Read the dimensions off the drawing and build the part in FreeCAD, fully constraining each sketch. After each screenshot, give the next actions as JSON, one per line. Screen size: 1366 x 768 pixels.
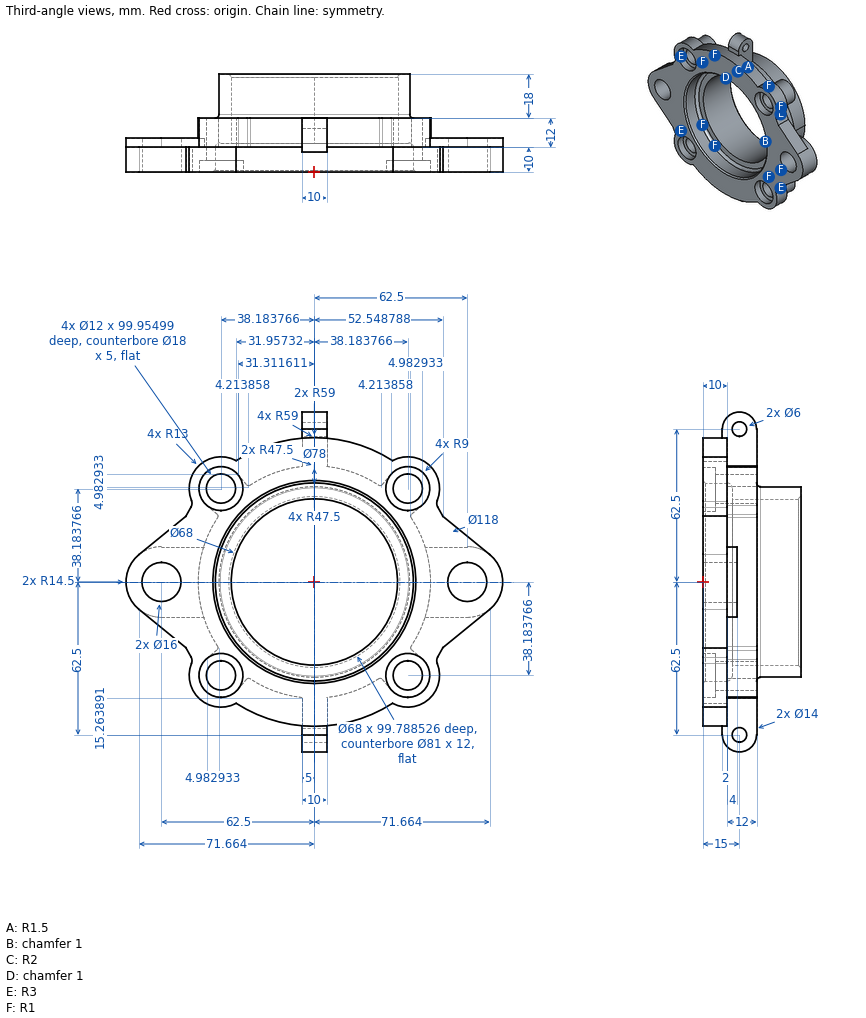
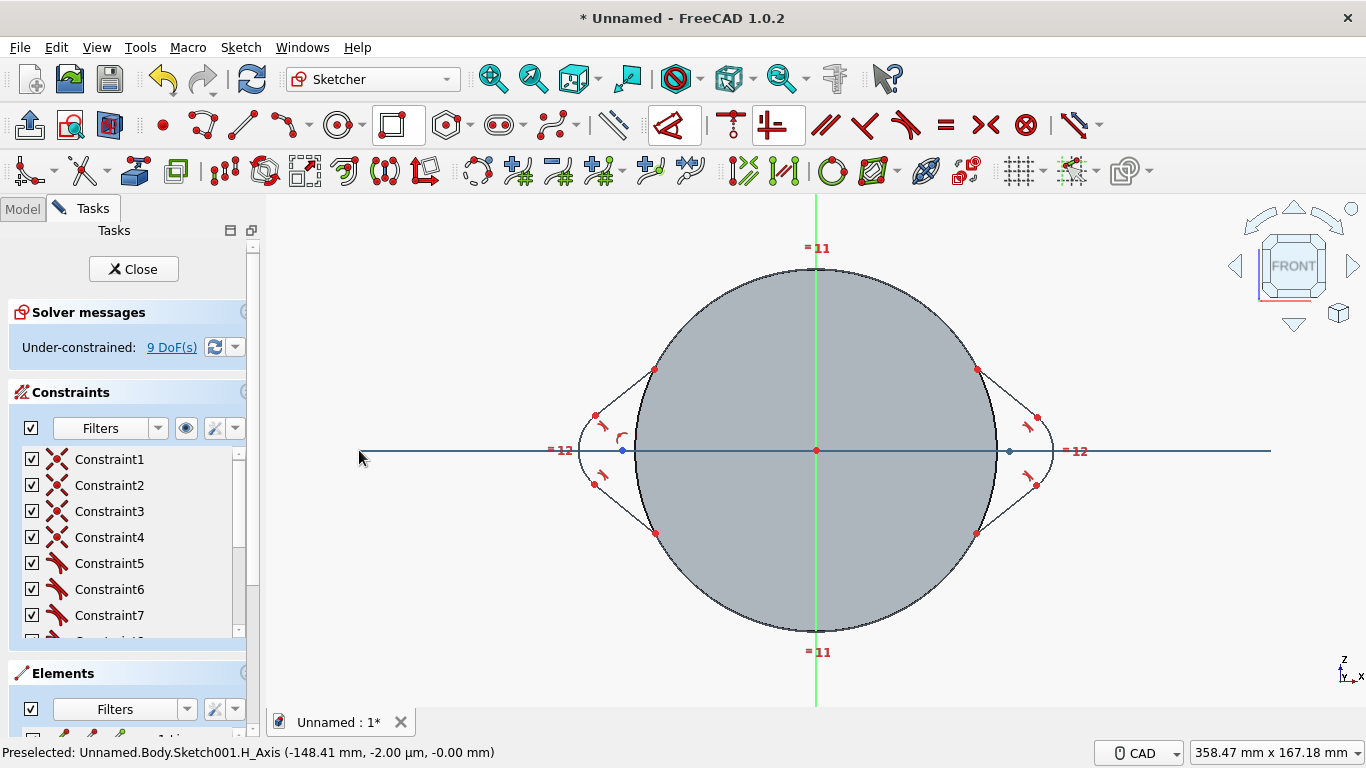
{"action": "left_click", "coordinate": [732, 126]}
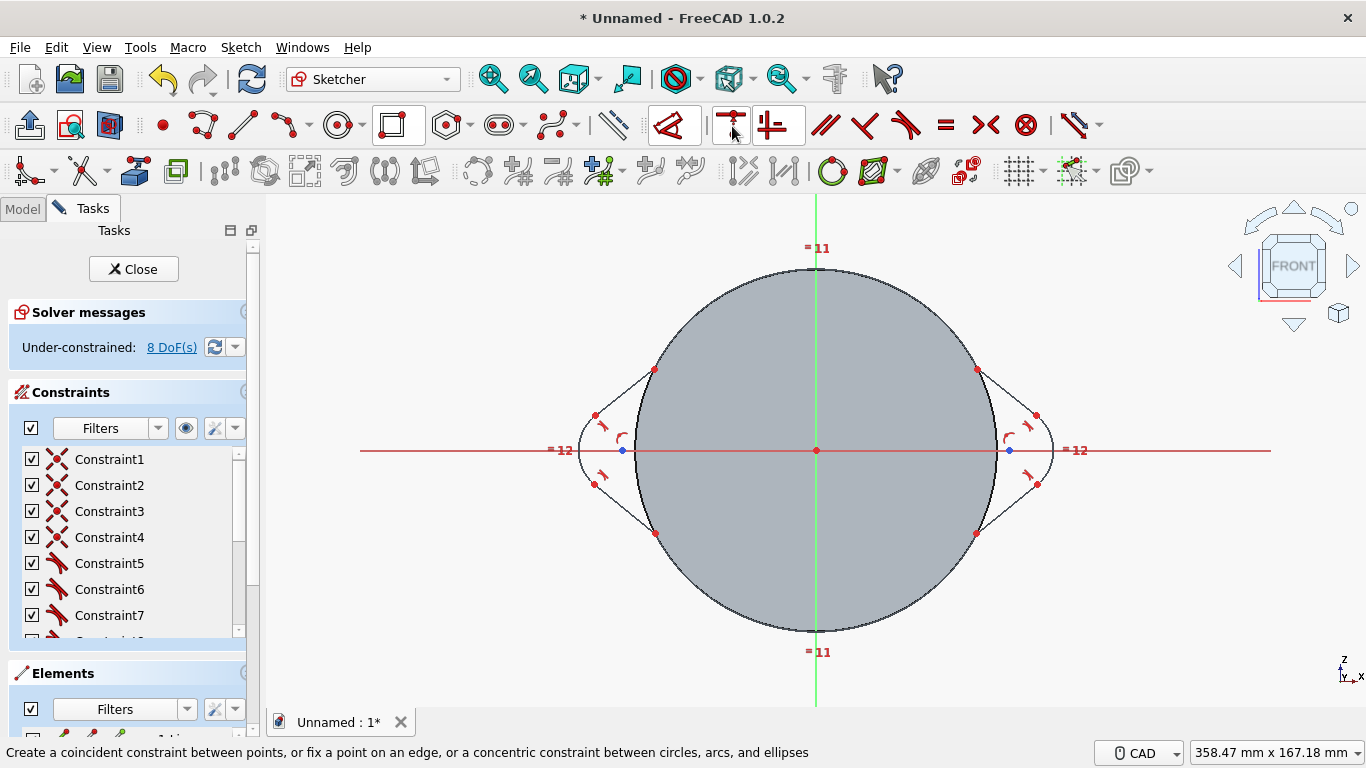
{"action": "left_click", "coordinate": [1037, 416]}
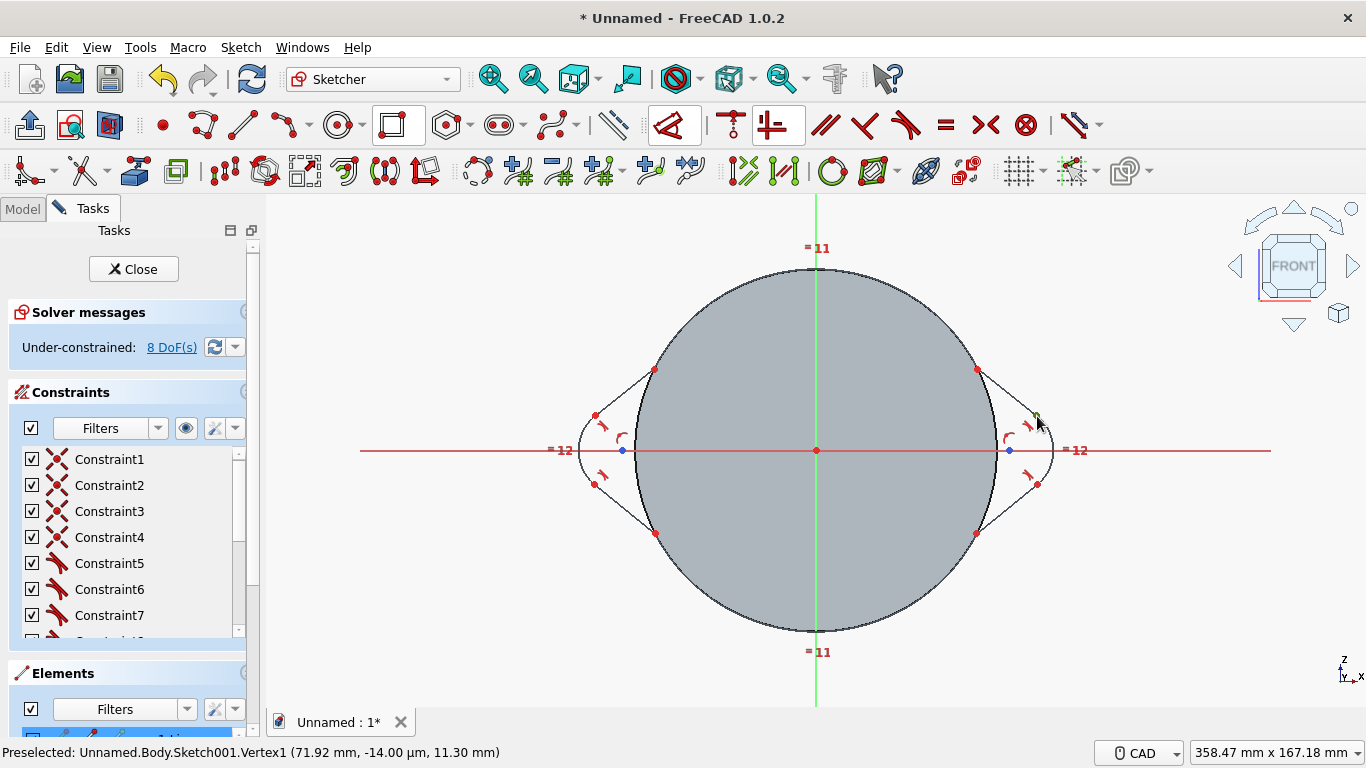
{"action": "left_click", "coordinate": [595, 416]}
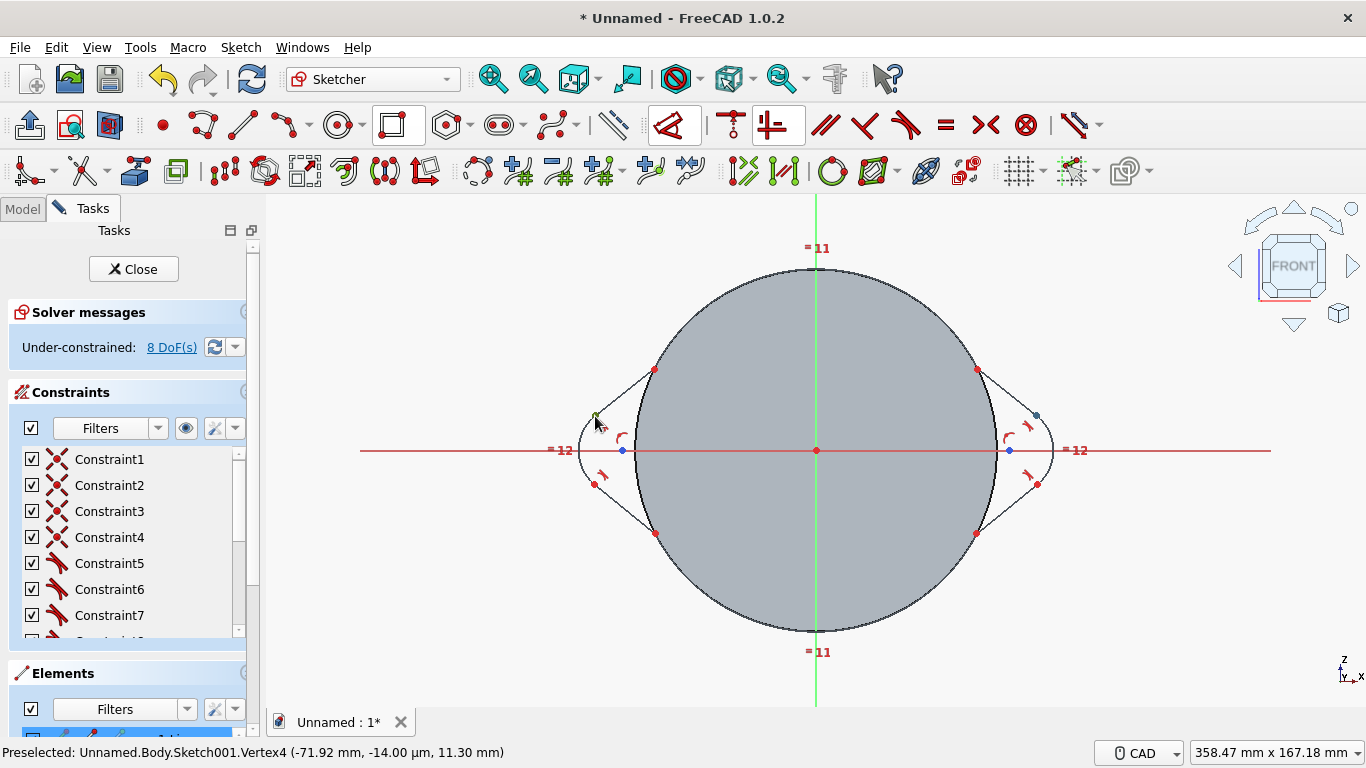
{"action": "left_click", "coordinate": [816, 581]}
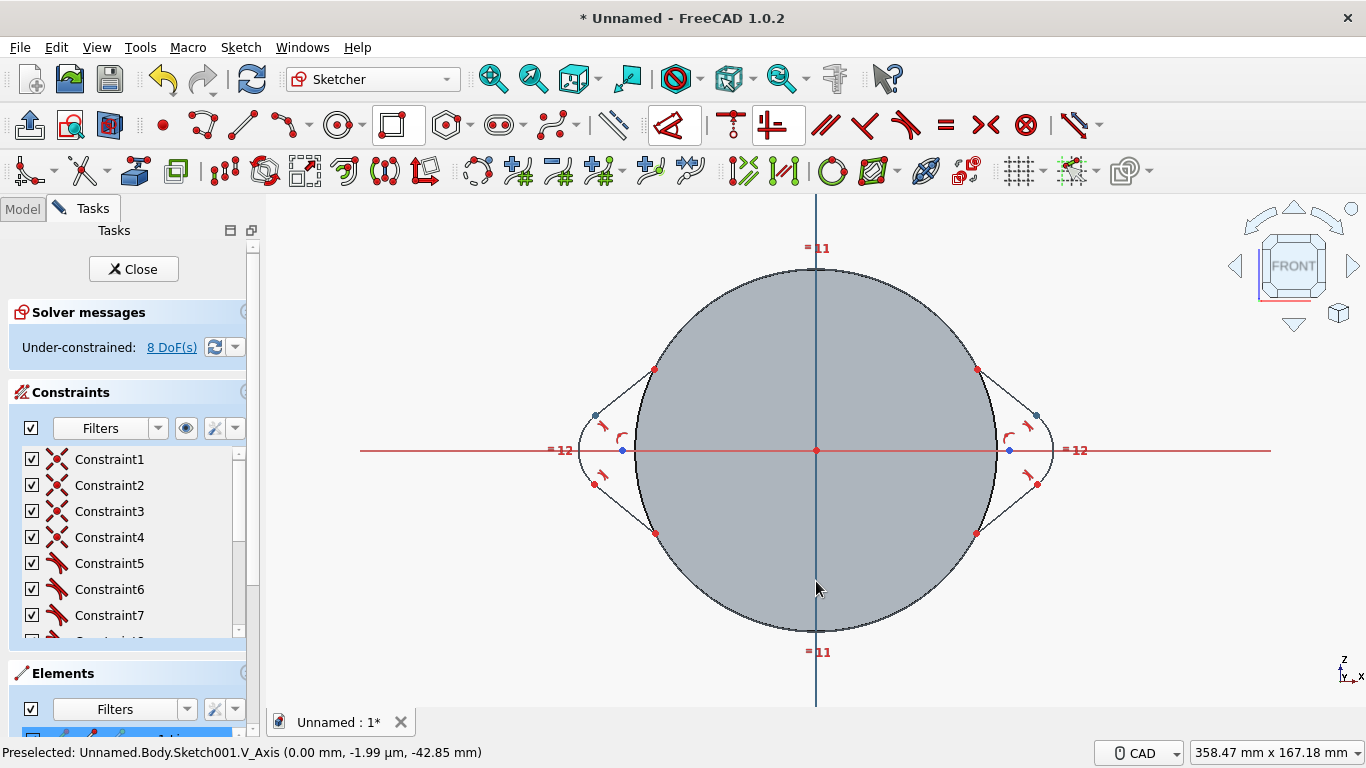
{"action": "left_click", "coordinate": [986, 126]}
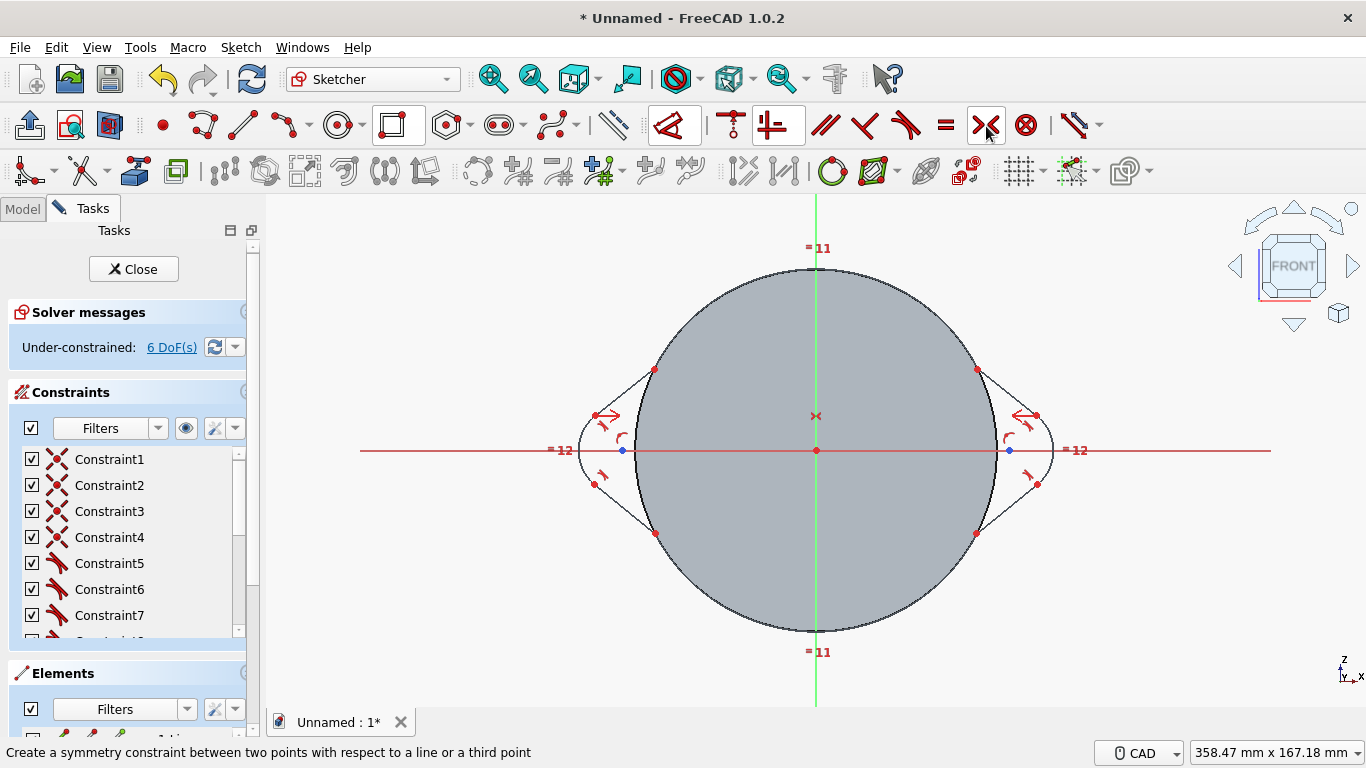
{"action": "left_click", "coordinate": [893, 287]}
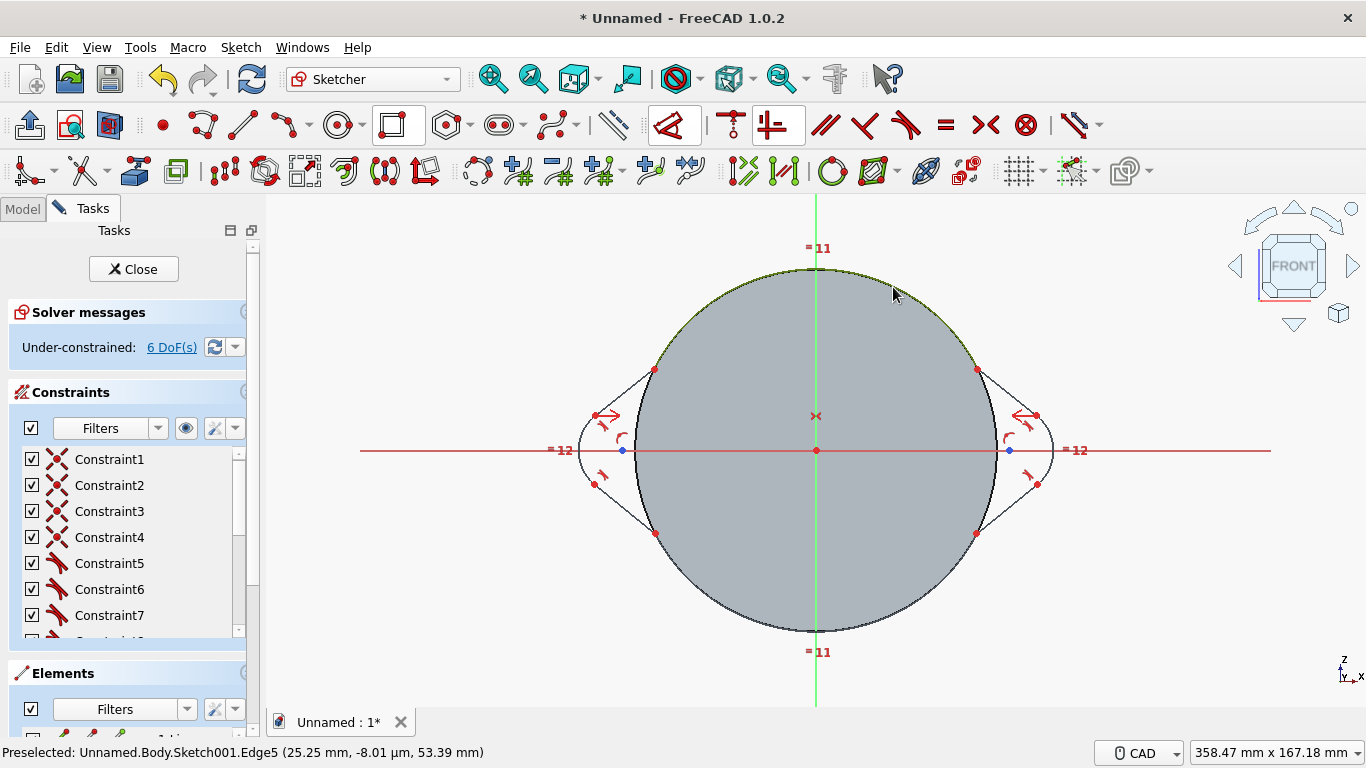
{"action": "left_click", "coordinate": [696, 126]}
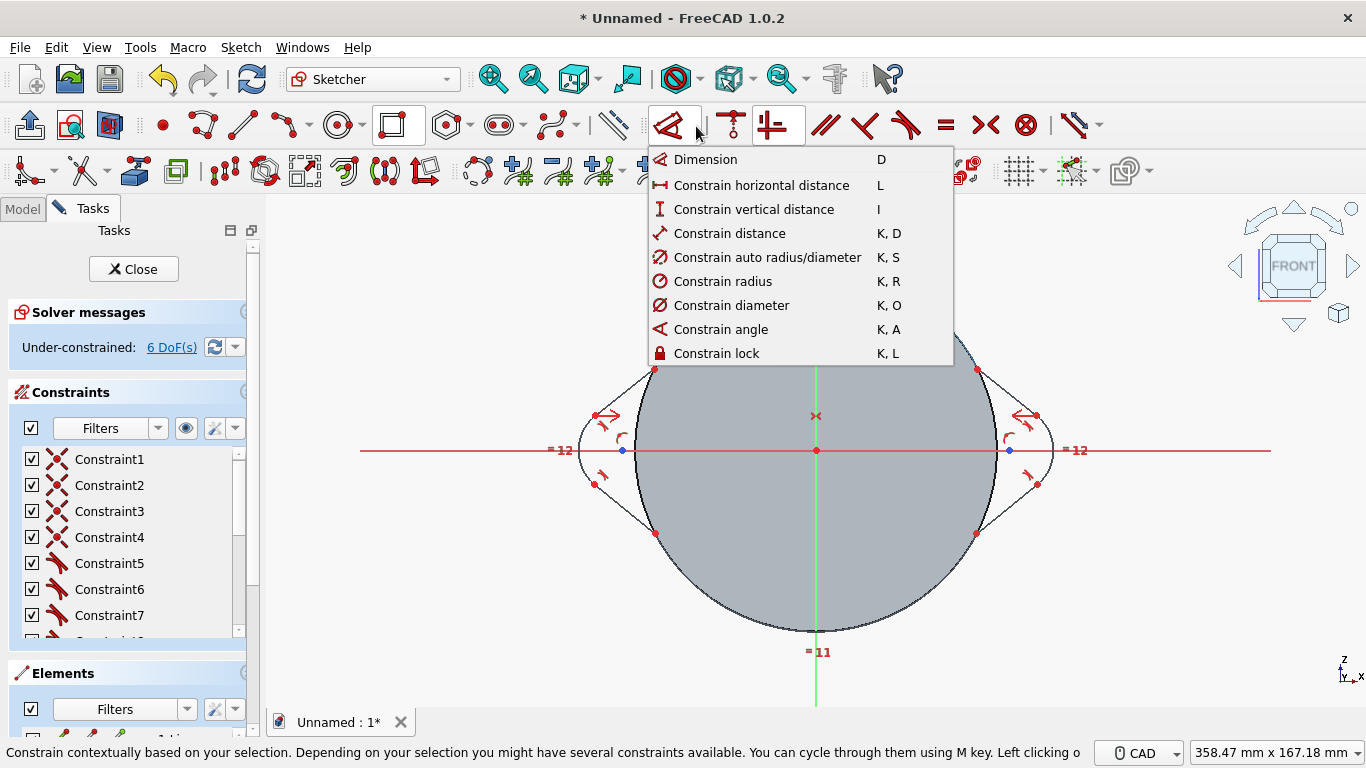
{"action": "left_click", "coordinate": [801, 281]}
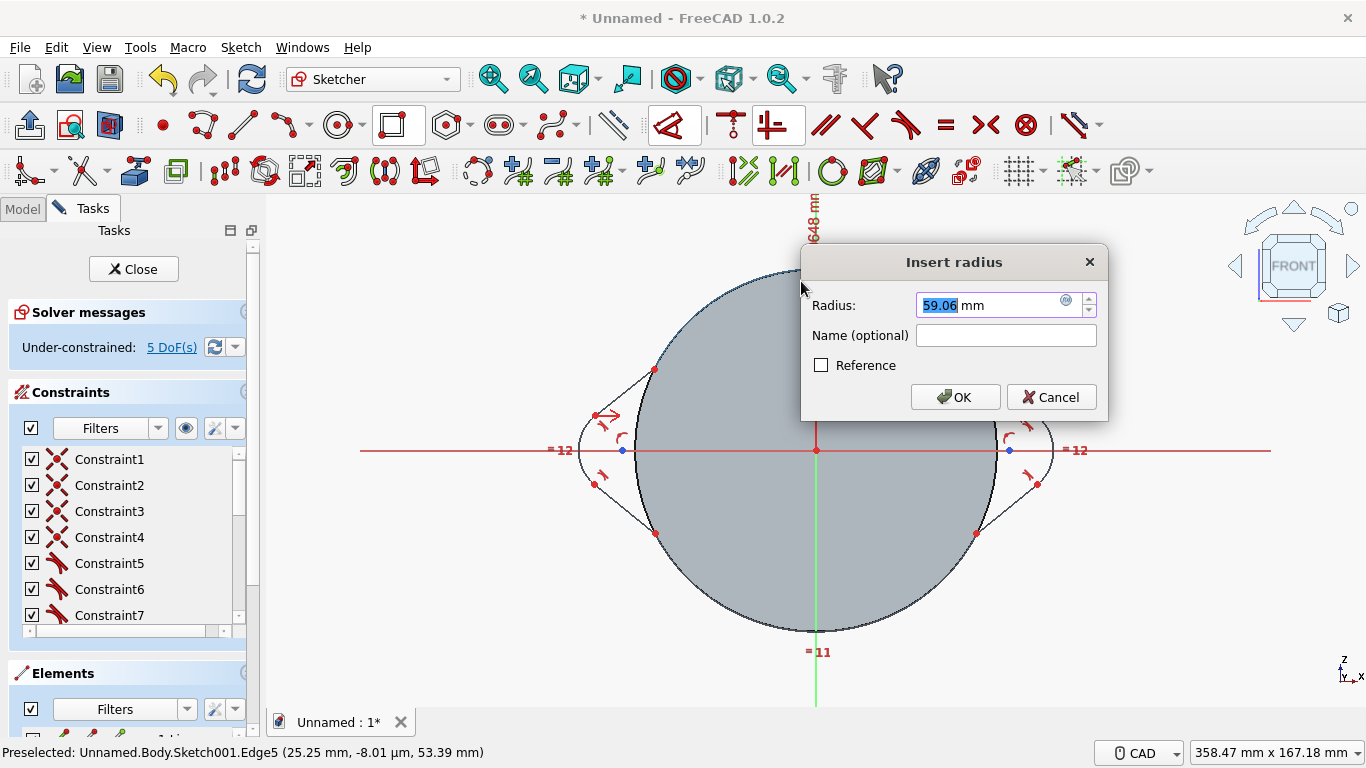
{"action": "type", "text": "59"}
{"action": "key", "text": "Return"}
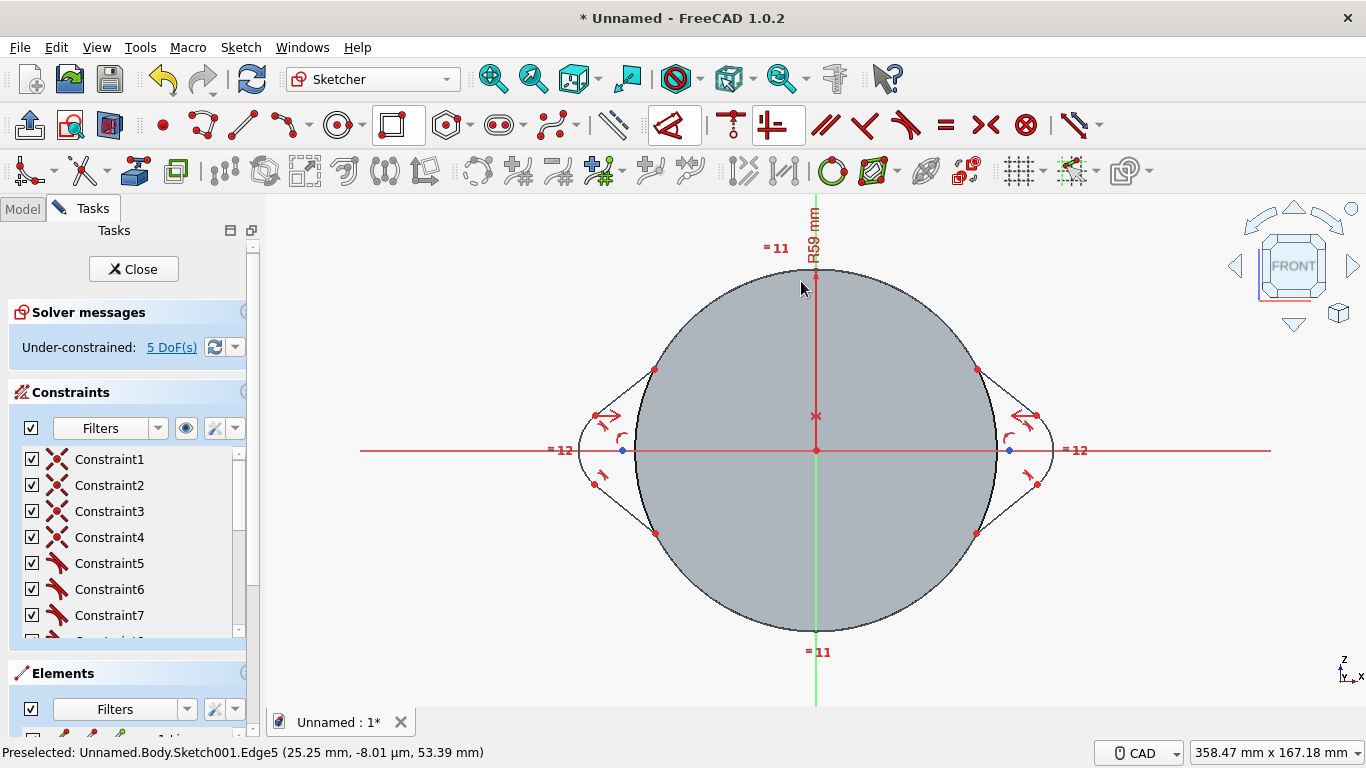
{"action": "left_click", "coordinate": [582, 435]}